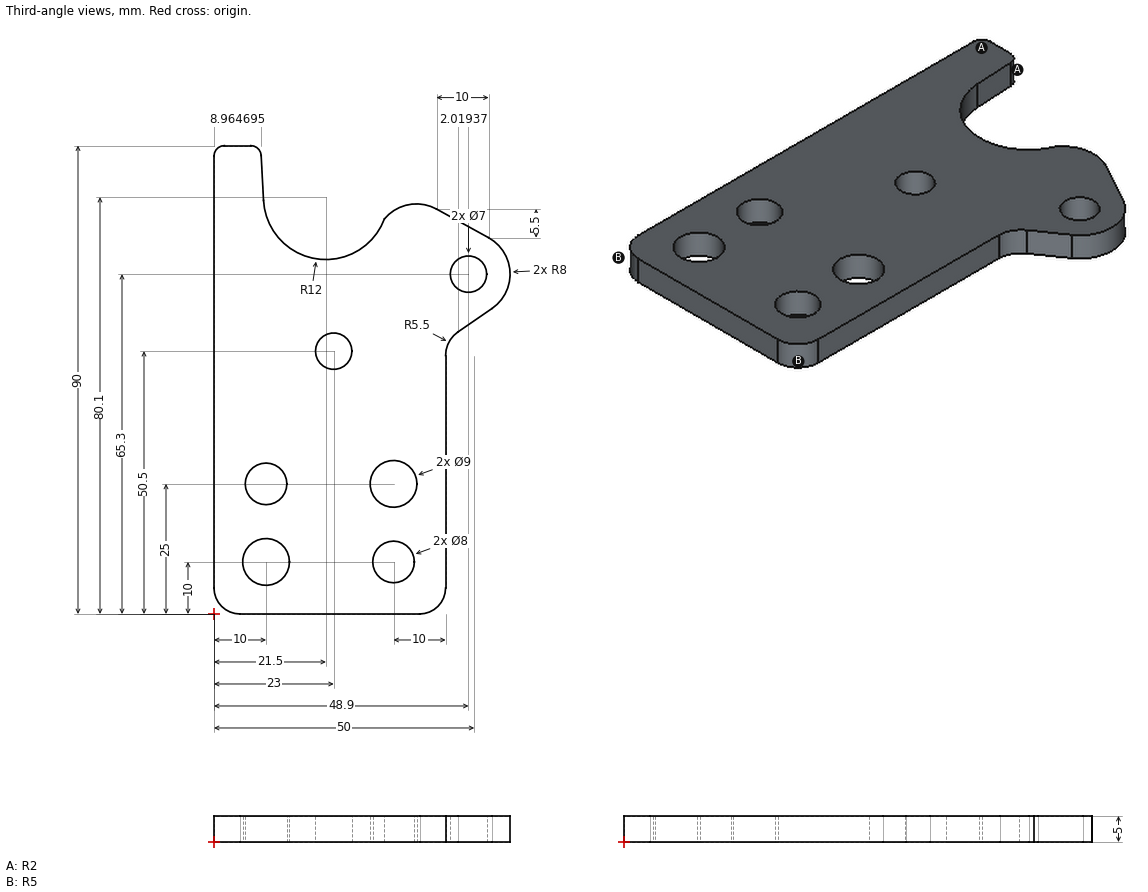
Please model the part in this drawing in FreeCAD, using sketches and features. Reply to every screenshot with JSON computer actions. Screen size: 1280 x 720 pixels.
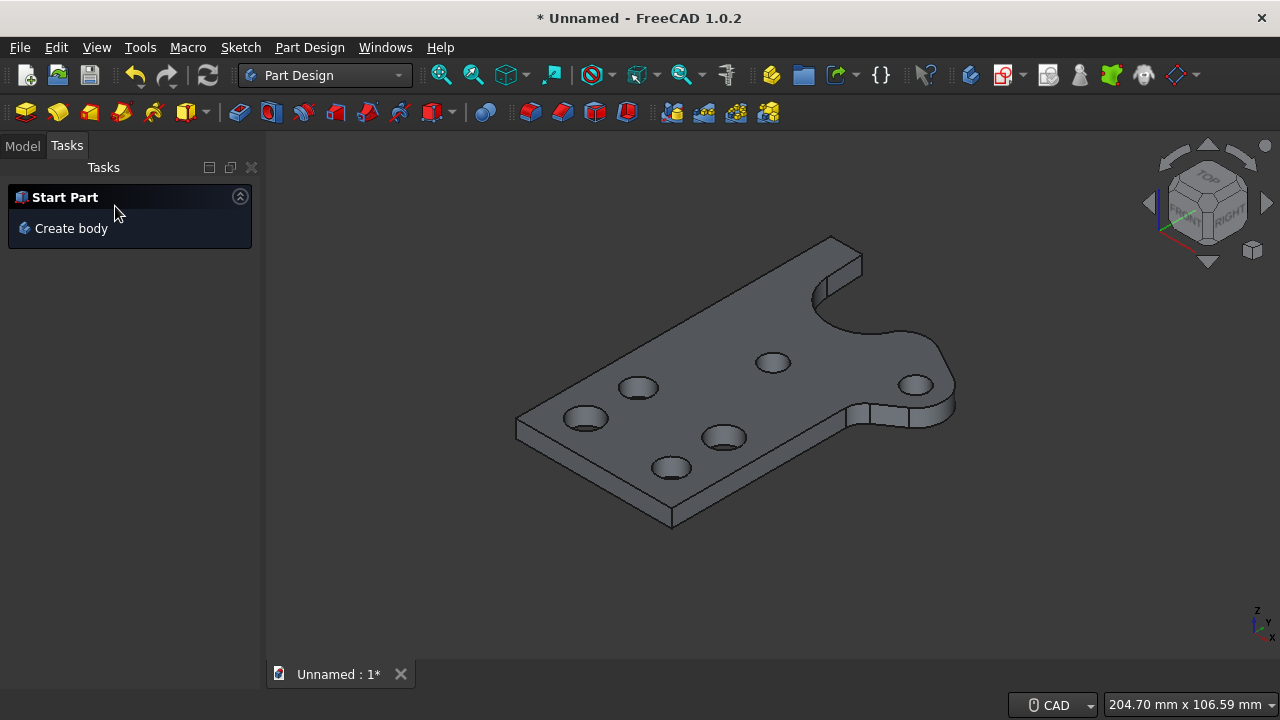
{"action": "key", "text": "2"}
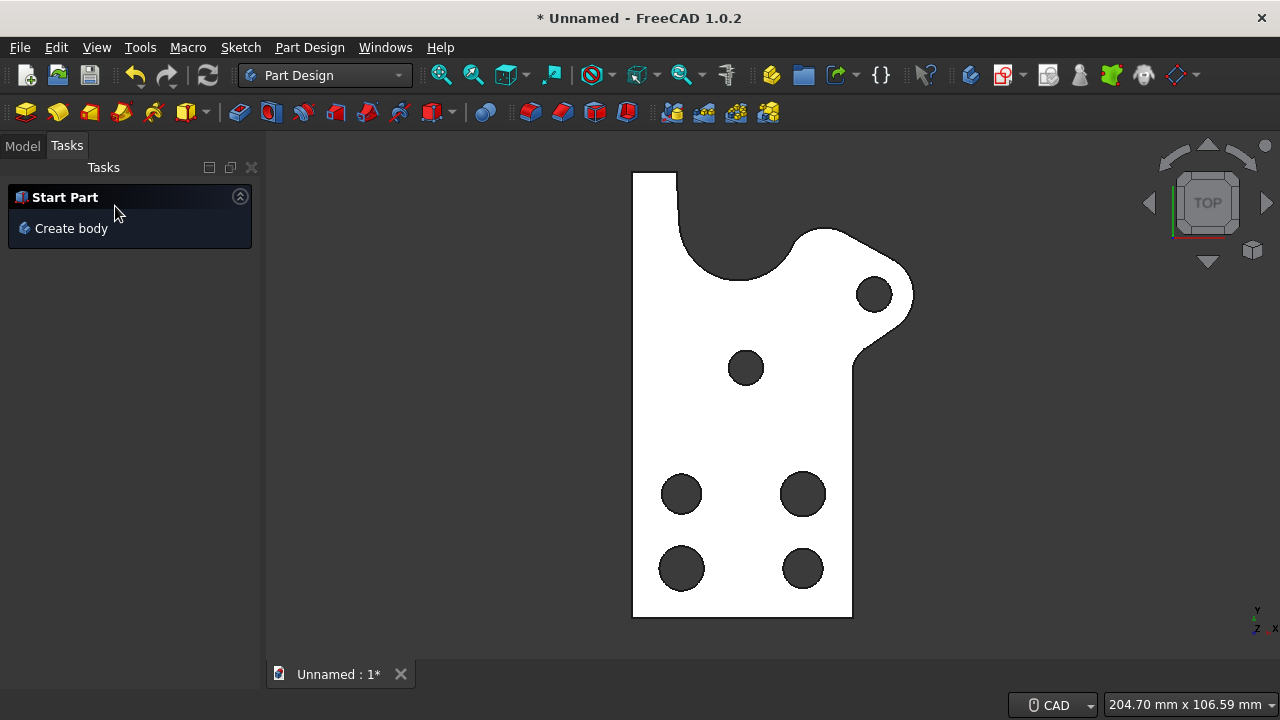
{"action": "key", "text": "1"}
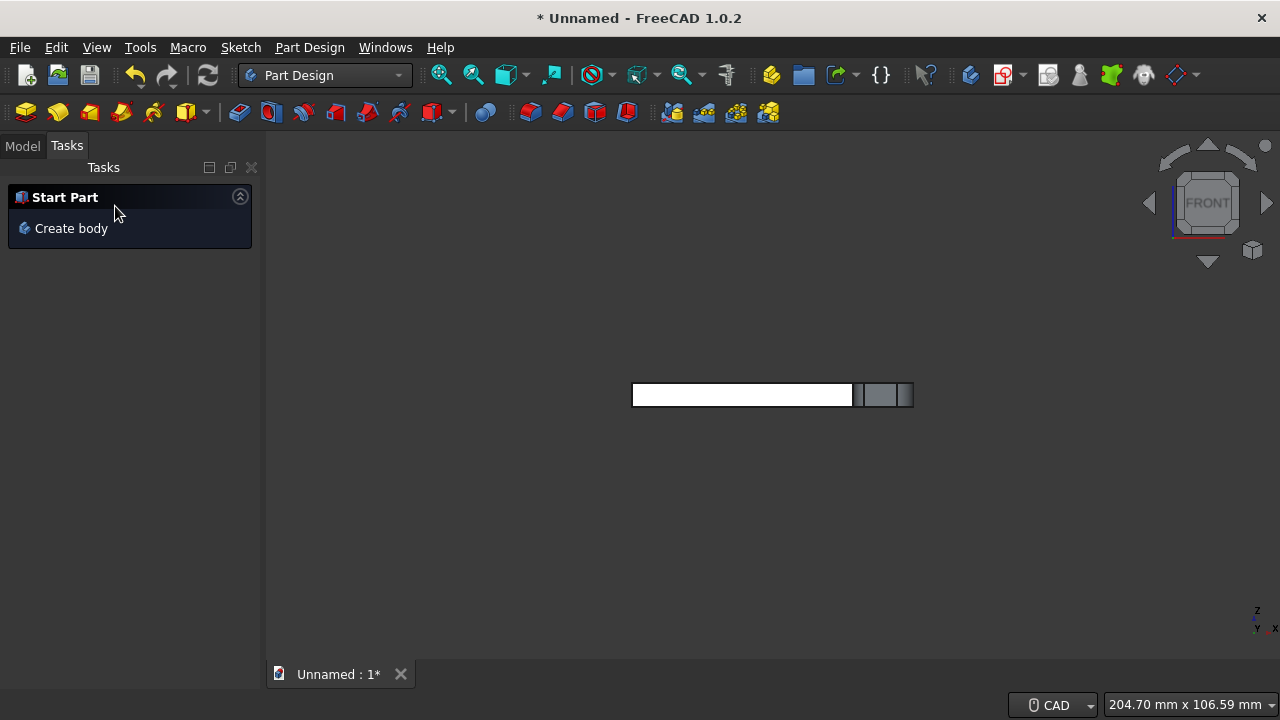
{"action": "key", "text": "v f"}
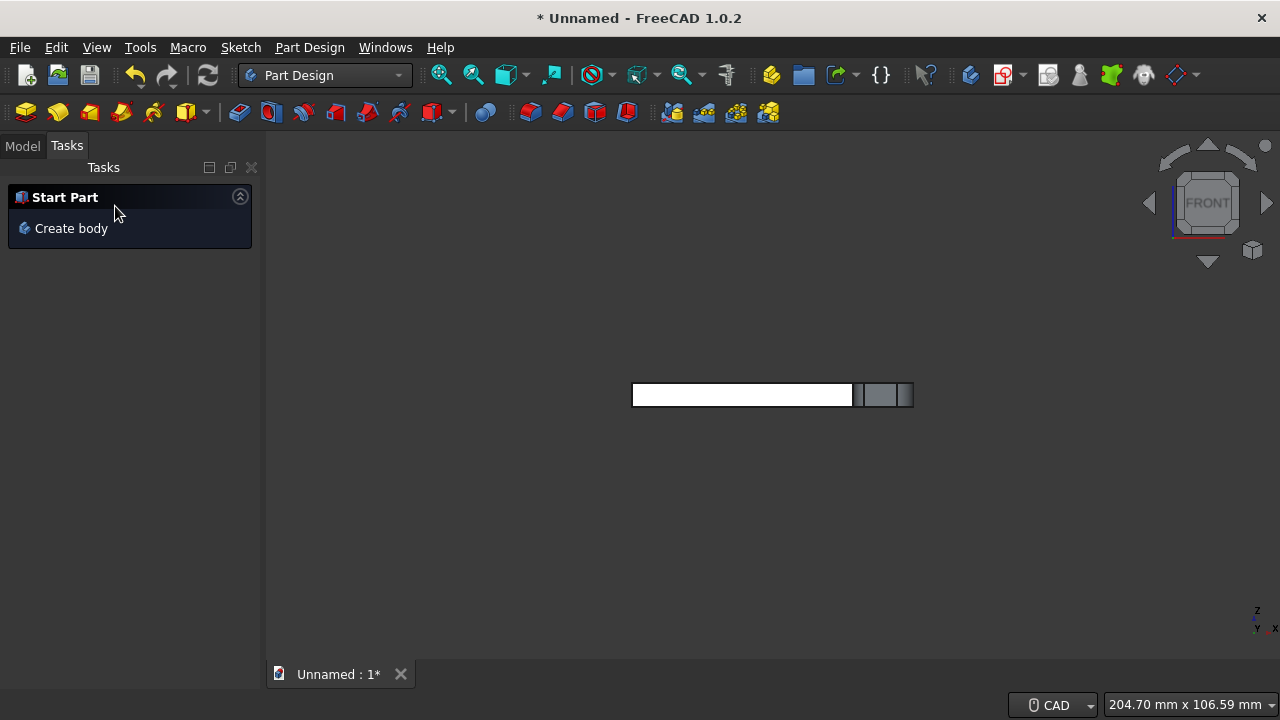
{"action": "key", "text": "3"}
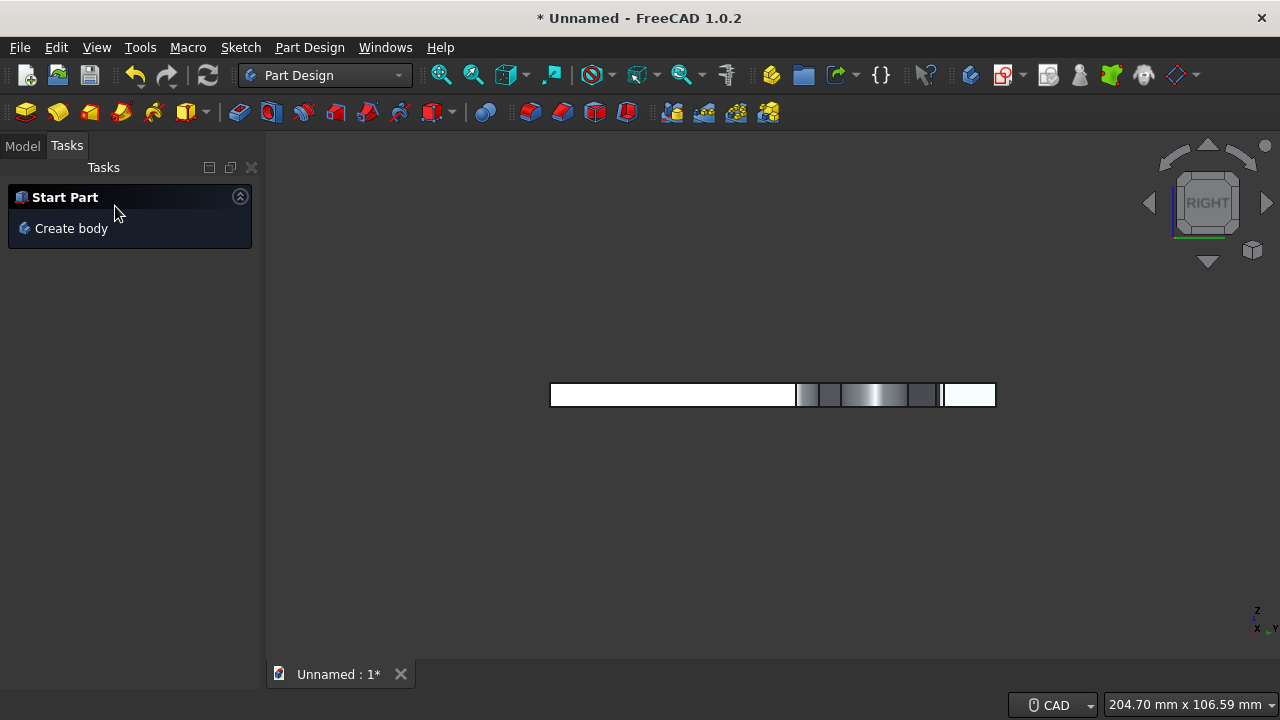
{"action": "key", "text": "v f"}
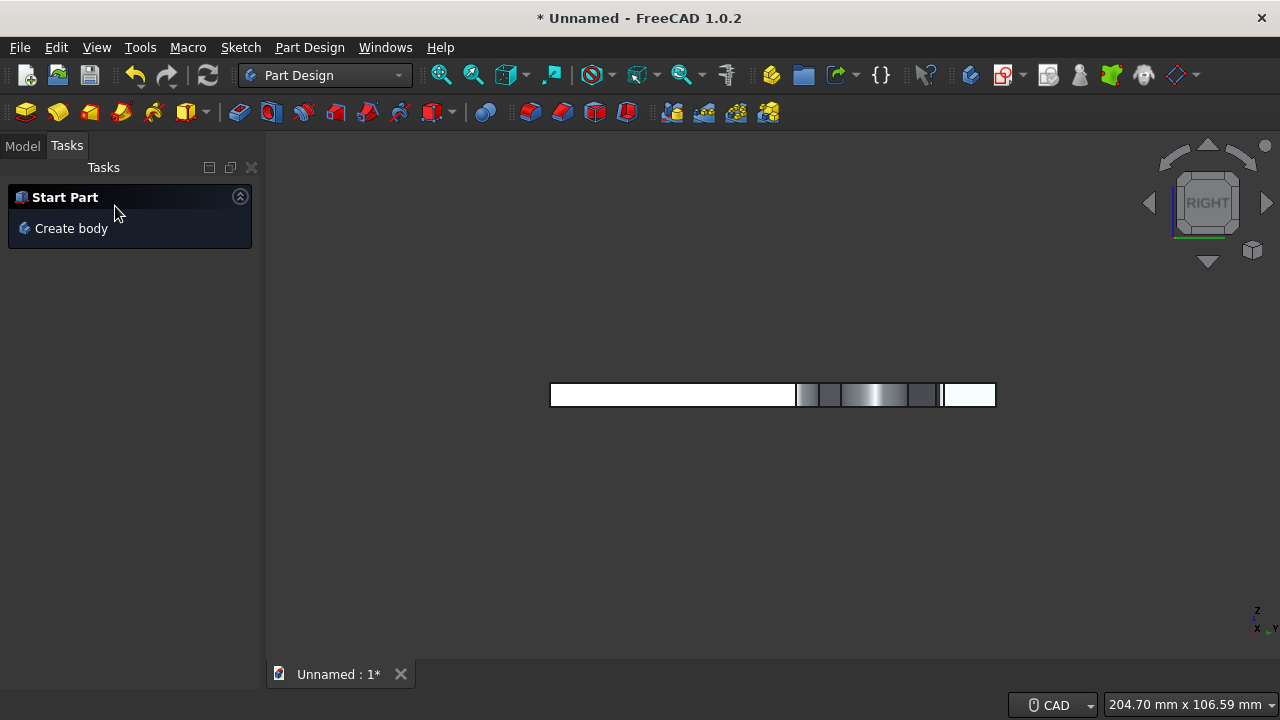
{"action": "key", "text": "5"}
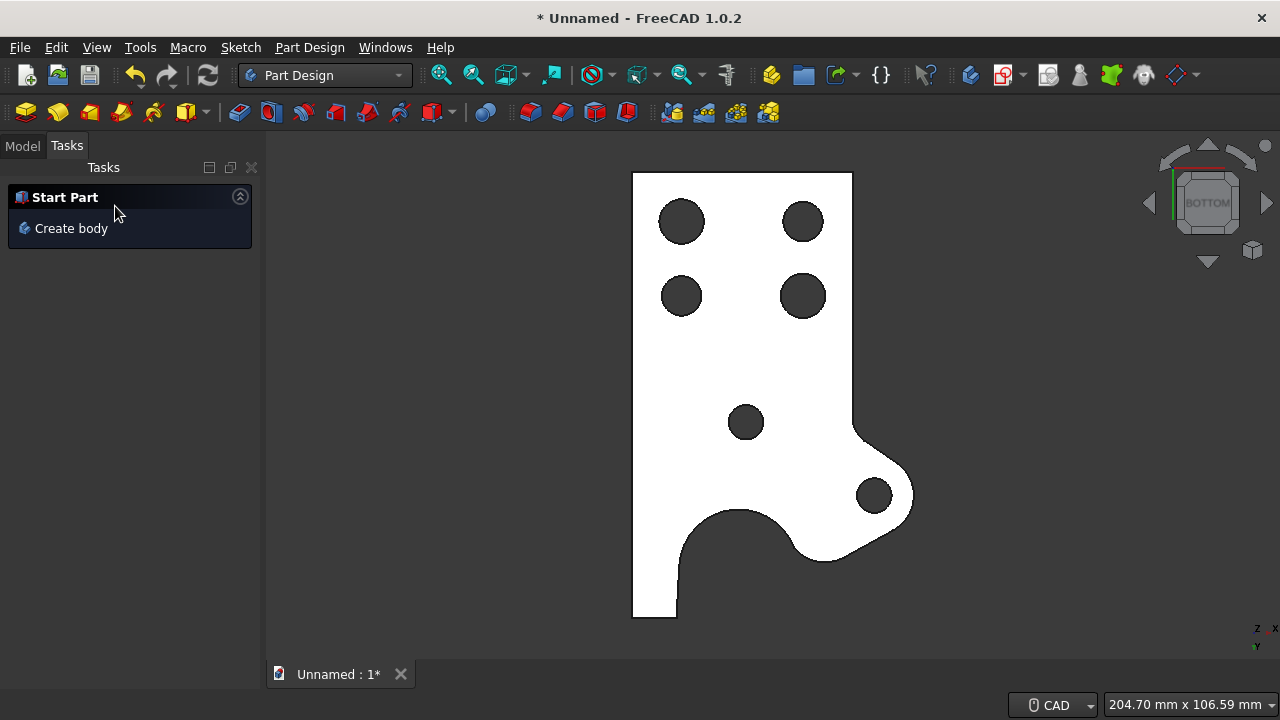
{"action": "key", "text": "4"}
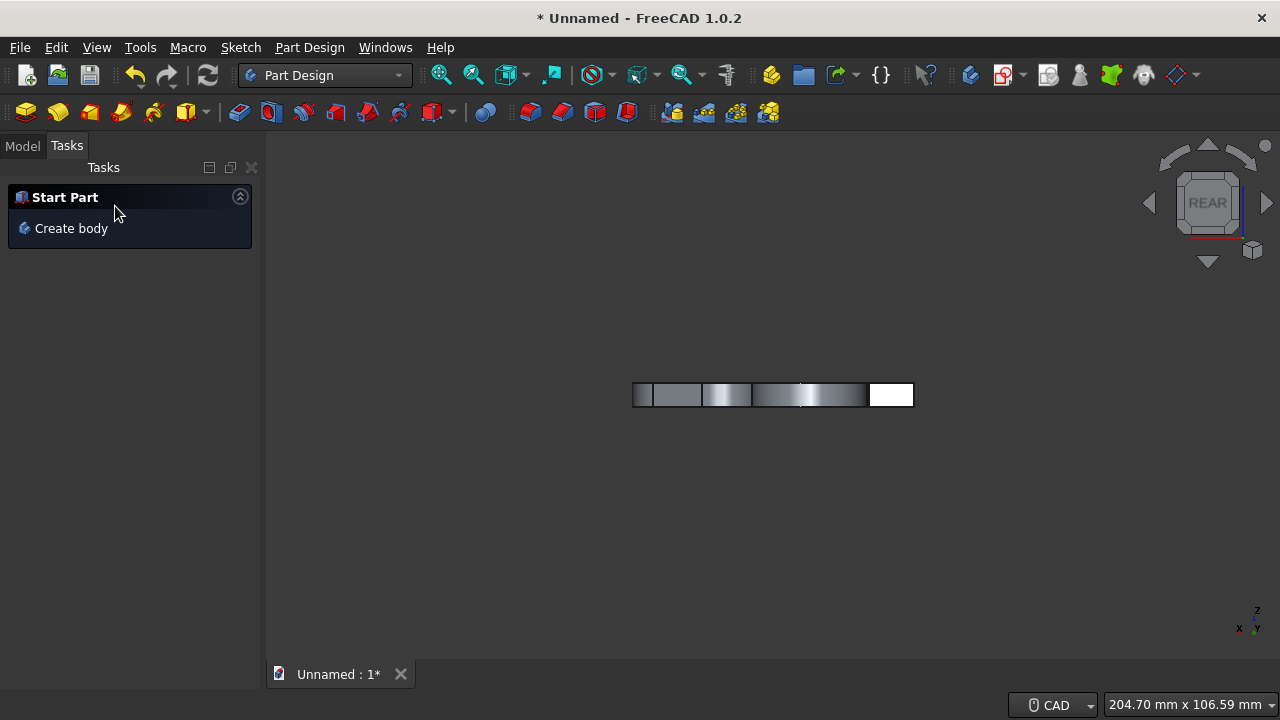
{"action": "key", "text": "v f"}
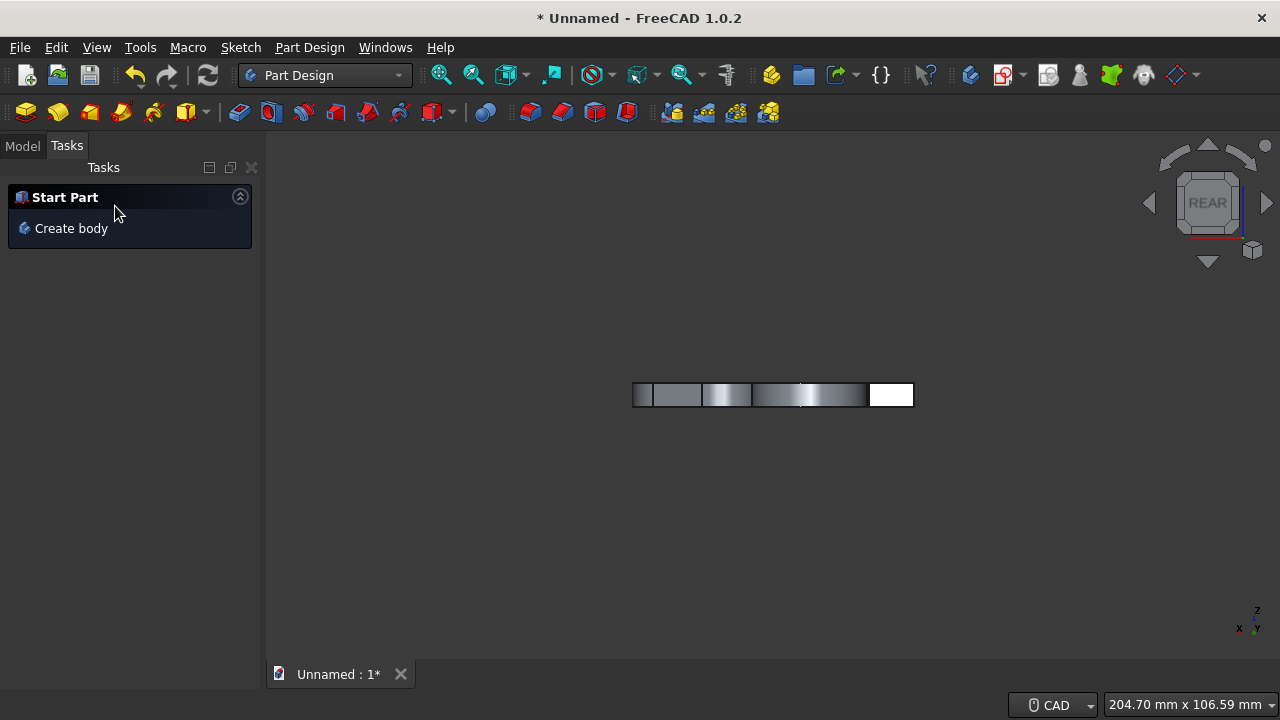
{"action": "left_click", "coordinate": [914, 394]}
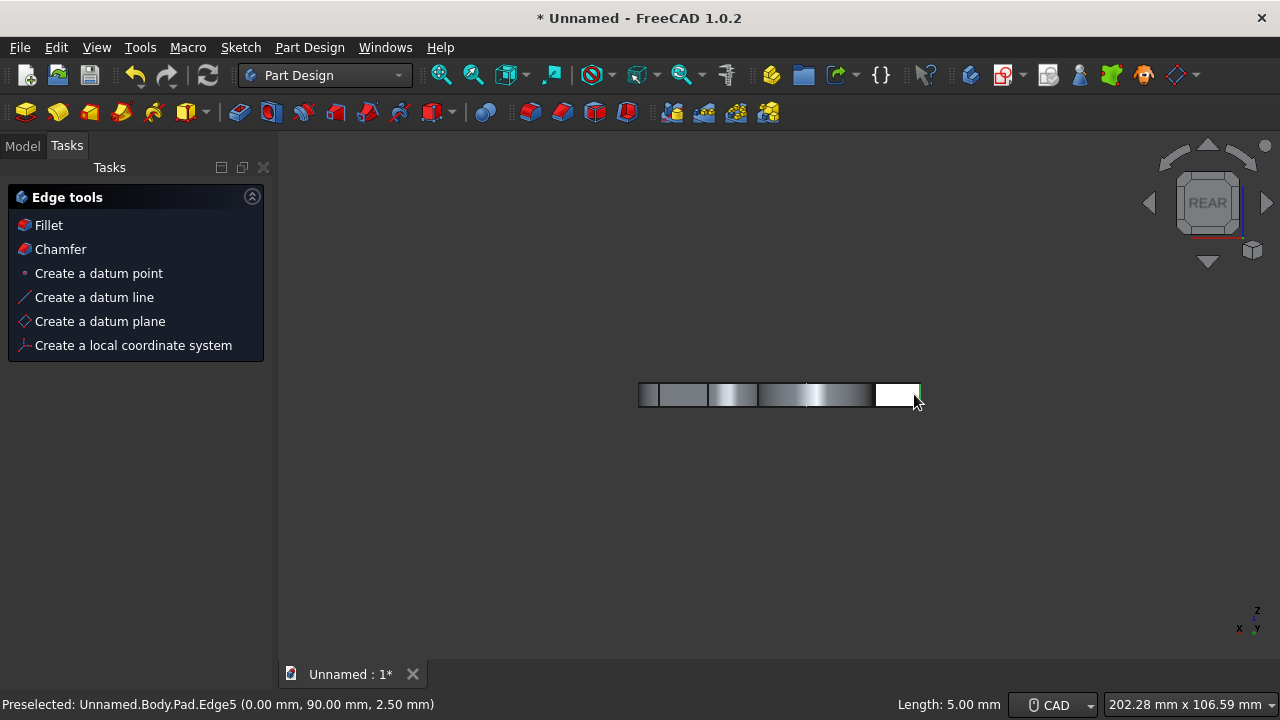
{"action": "left_click", "coordinate": [875, 394], "text": "ctrl"}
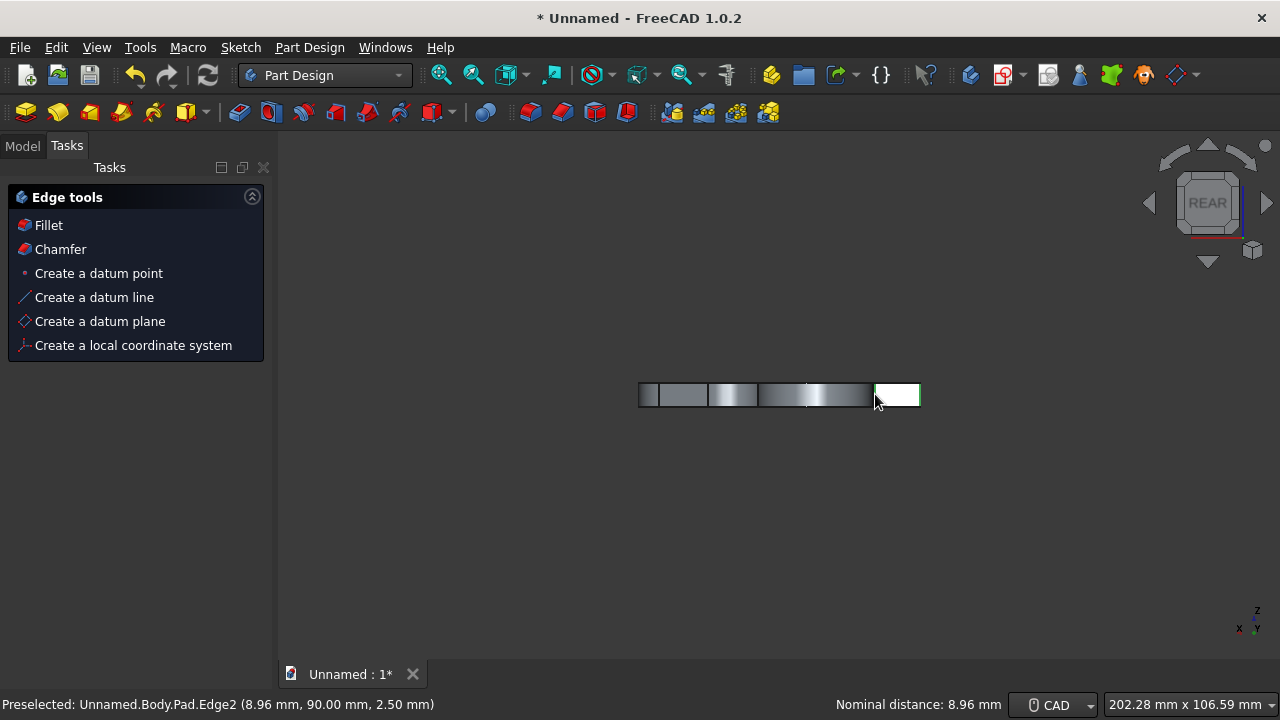
{"action": "left_click", "coordinate": [532, 112]}